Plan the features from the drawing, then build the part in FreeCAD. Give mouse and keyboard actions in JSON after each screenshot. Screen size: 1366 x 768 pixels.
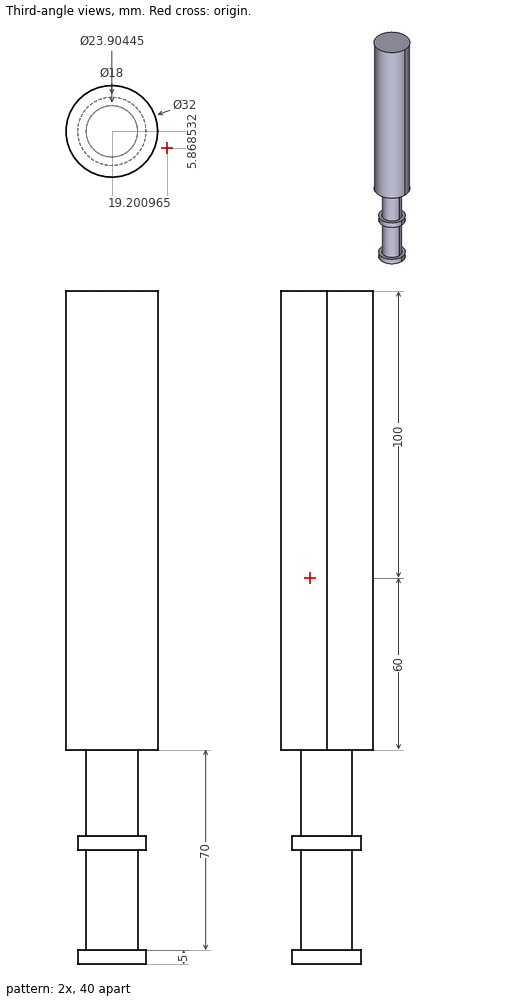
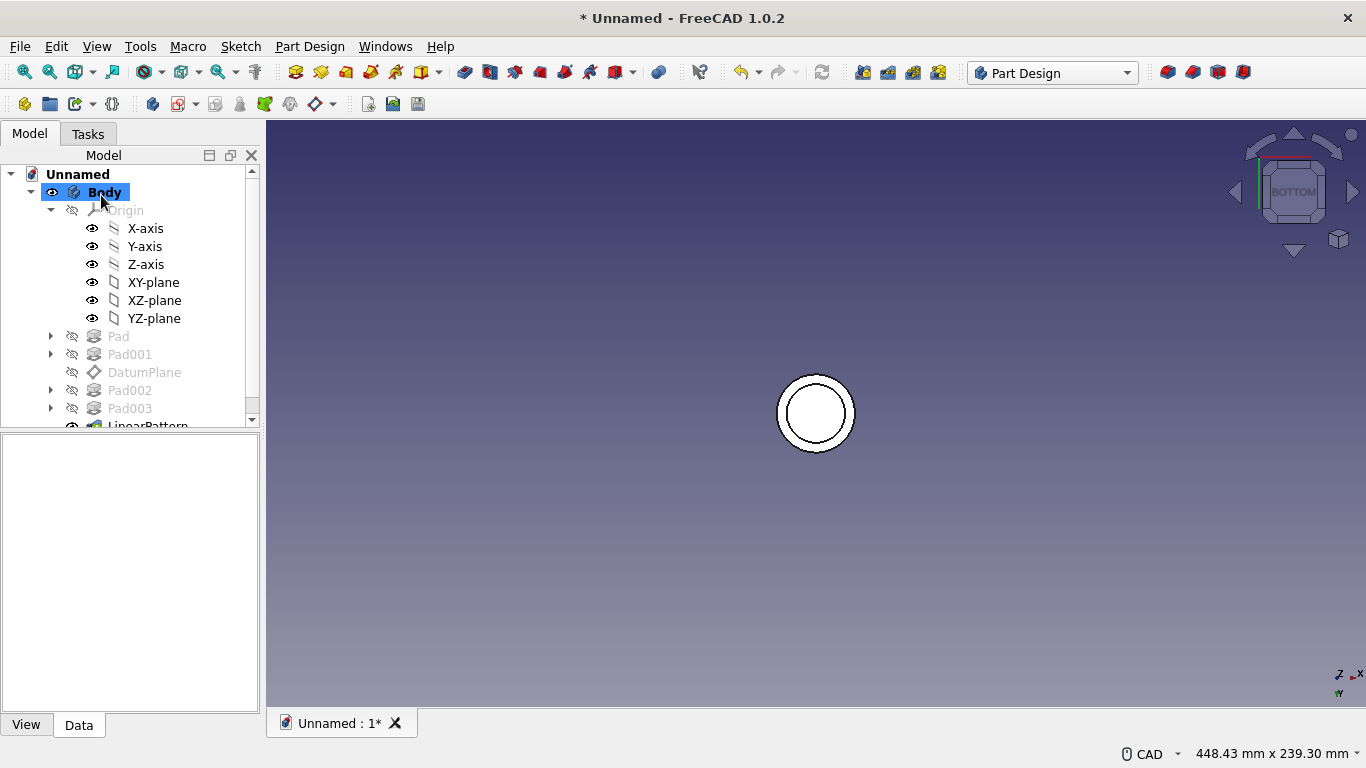
{"action": "key", "text": "0"}